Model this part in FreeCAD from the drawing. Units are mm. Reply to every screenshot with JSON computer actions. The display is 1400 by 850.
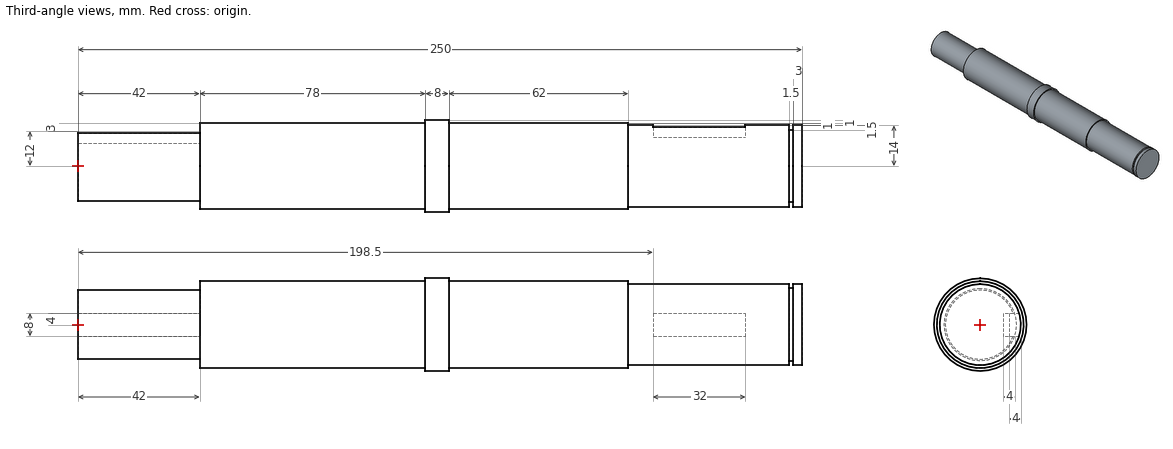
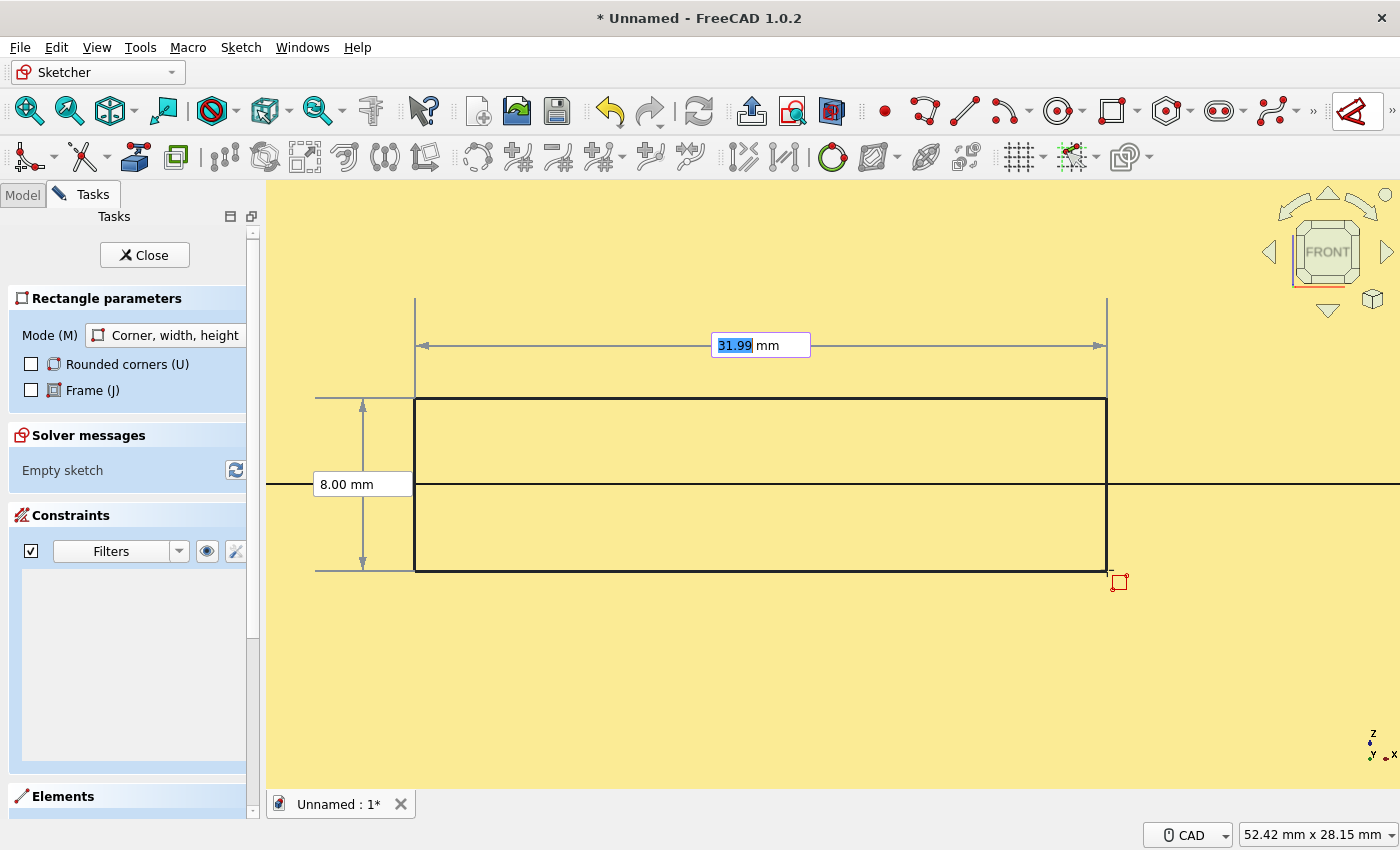
{"action": "type", "text": "32"}
{"action": "key", "text": "Tab"}
{"action": "type", "text": "8"}
{"action": "key", "text": "Return"}
{"action": "key", "text": "Escape"}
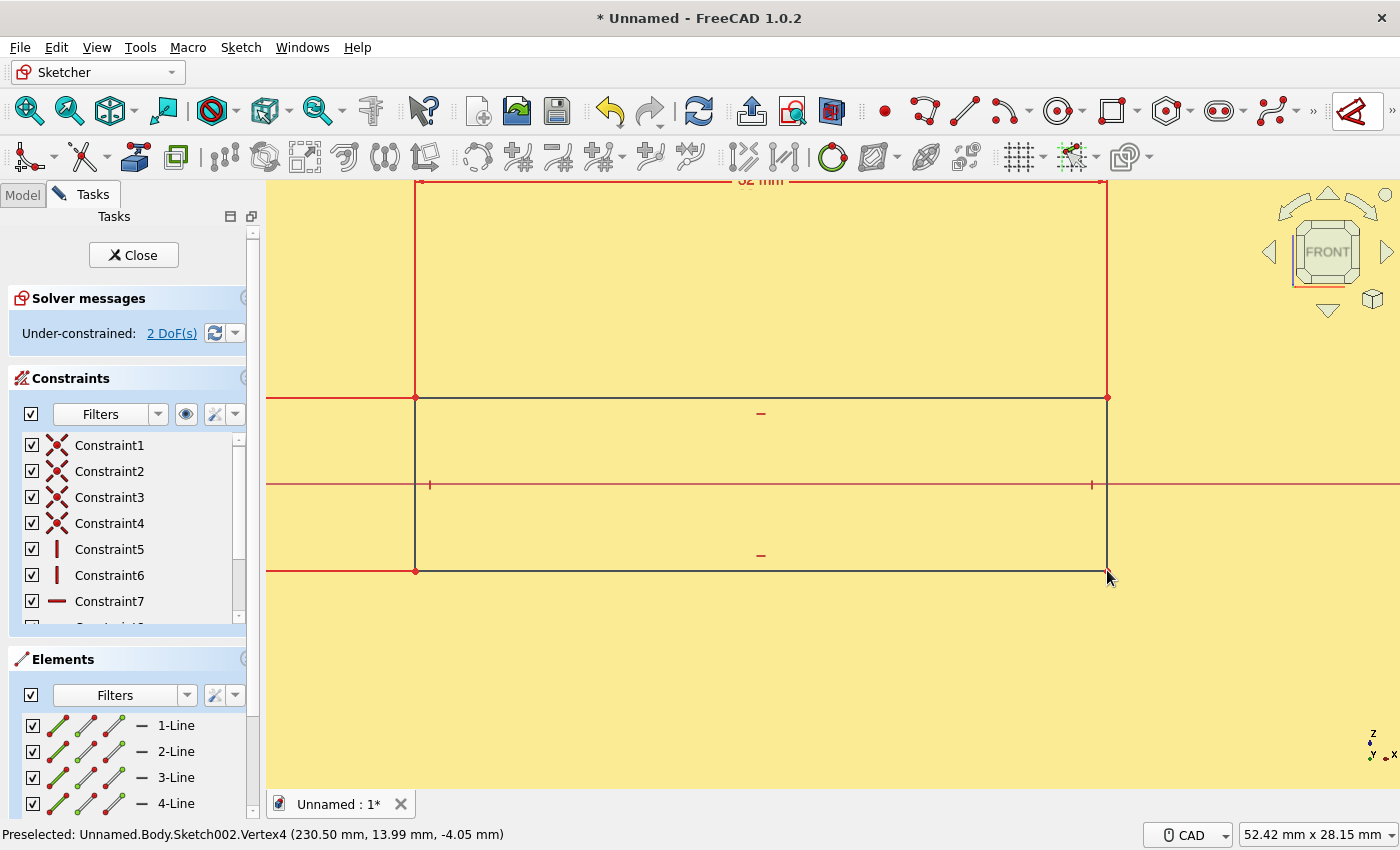
{"action": "left_click", "coordinate": [415, 398]}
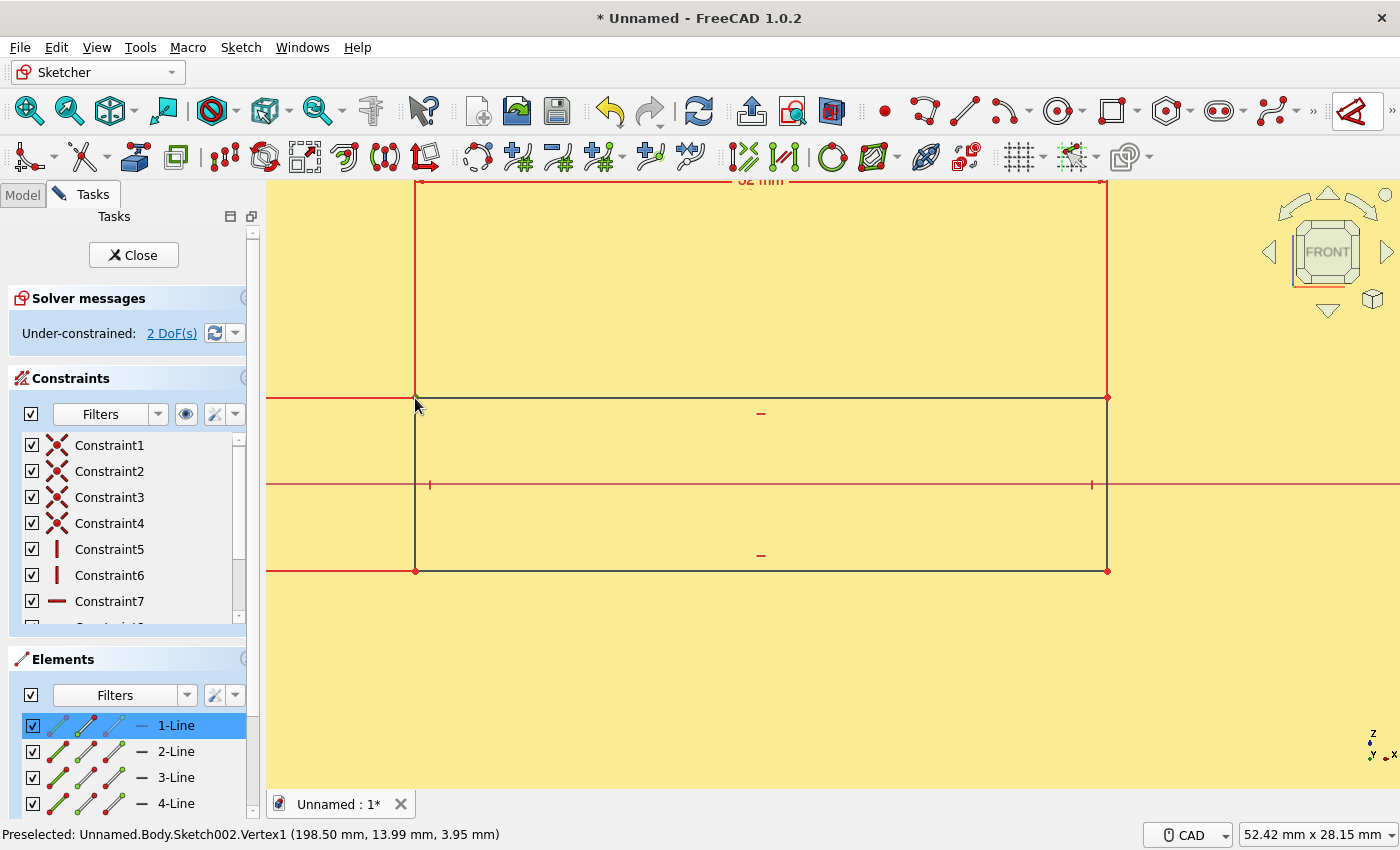
{"action": "left_click", "coordinate": [1378, 112]}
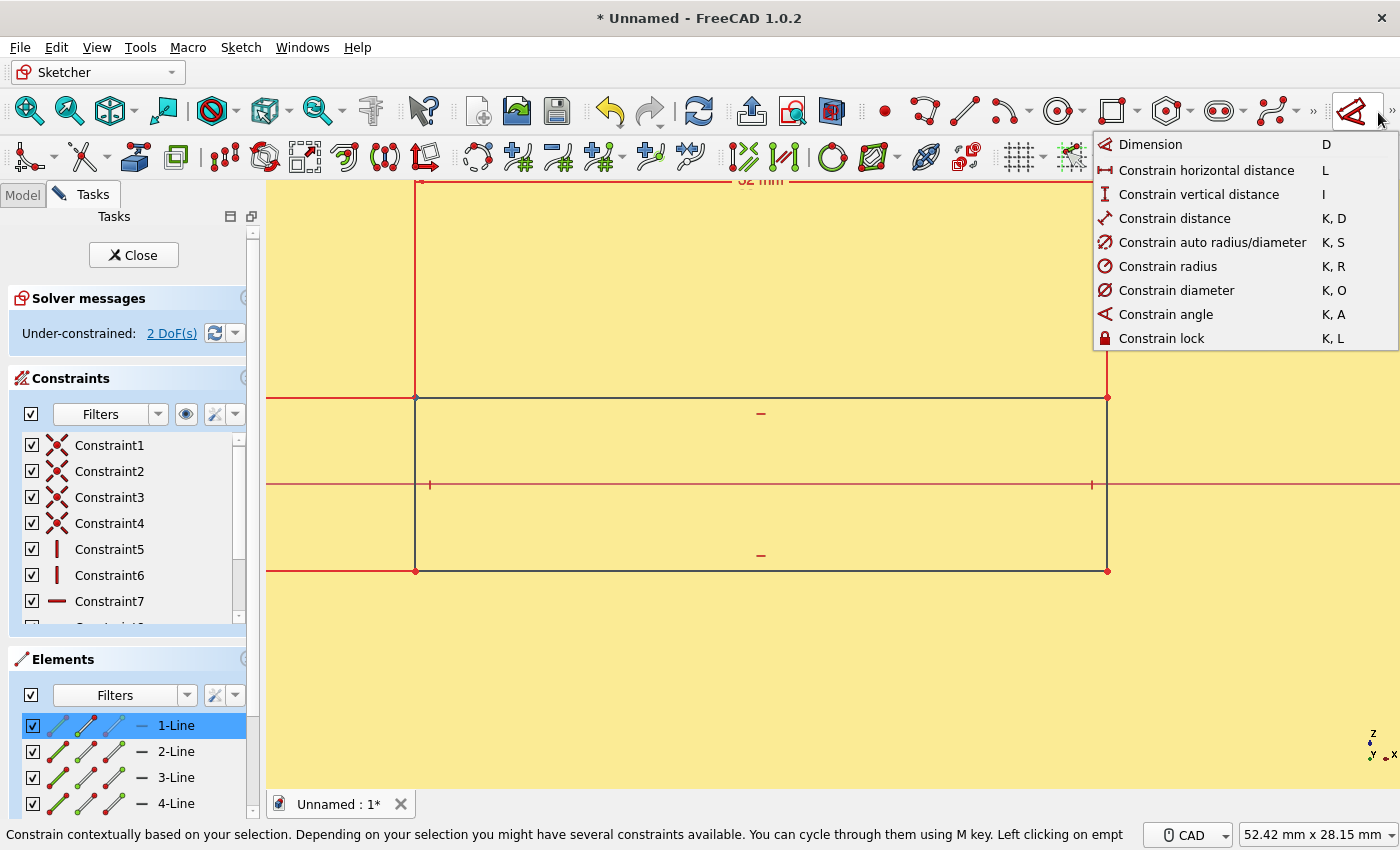
{"action": "left_click", "coordinate": [1246, 194]}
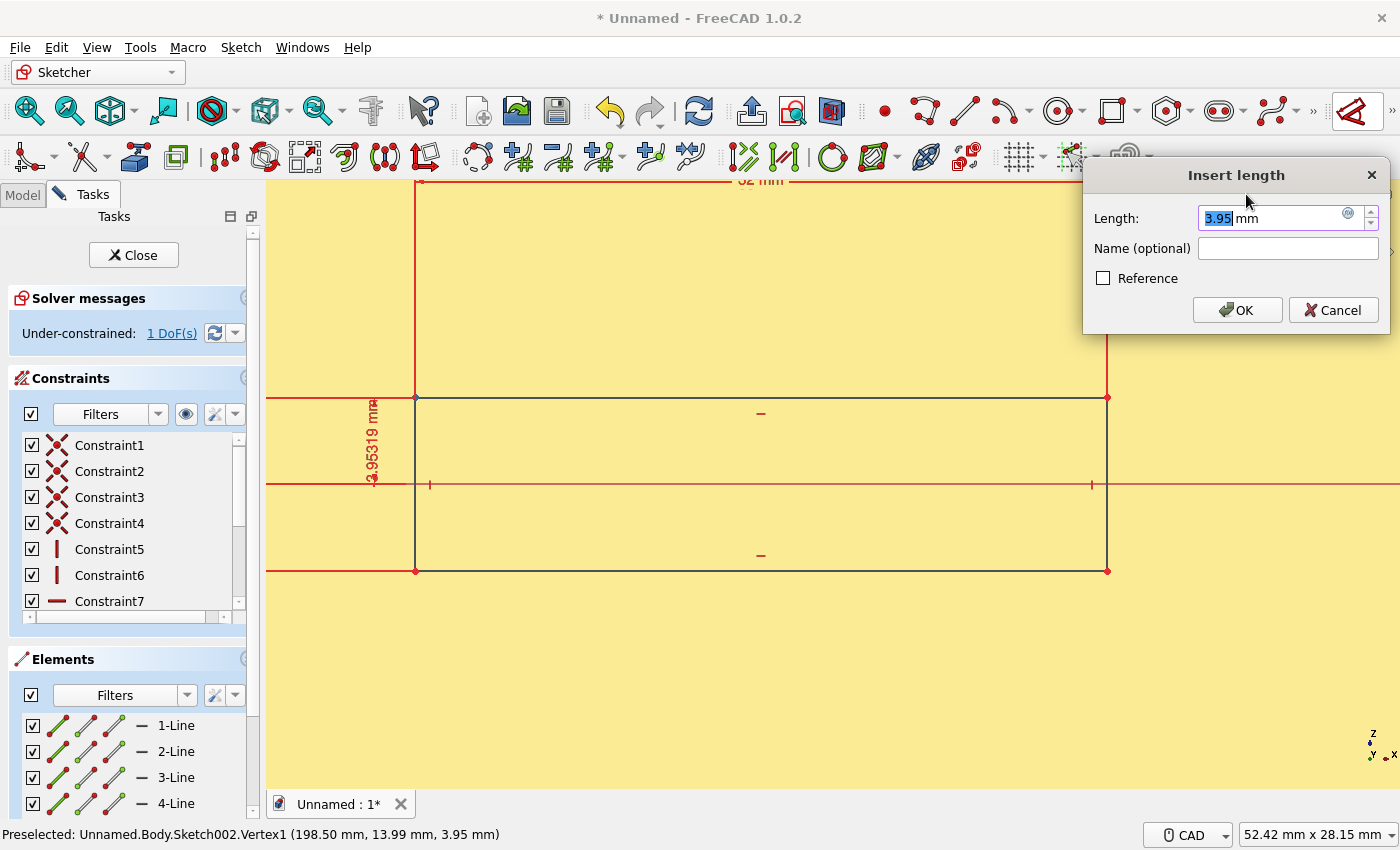
{"action": "type", "text": "4"}
{"action": "key", "text": "Return"}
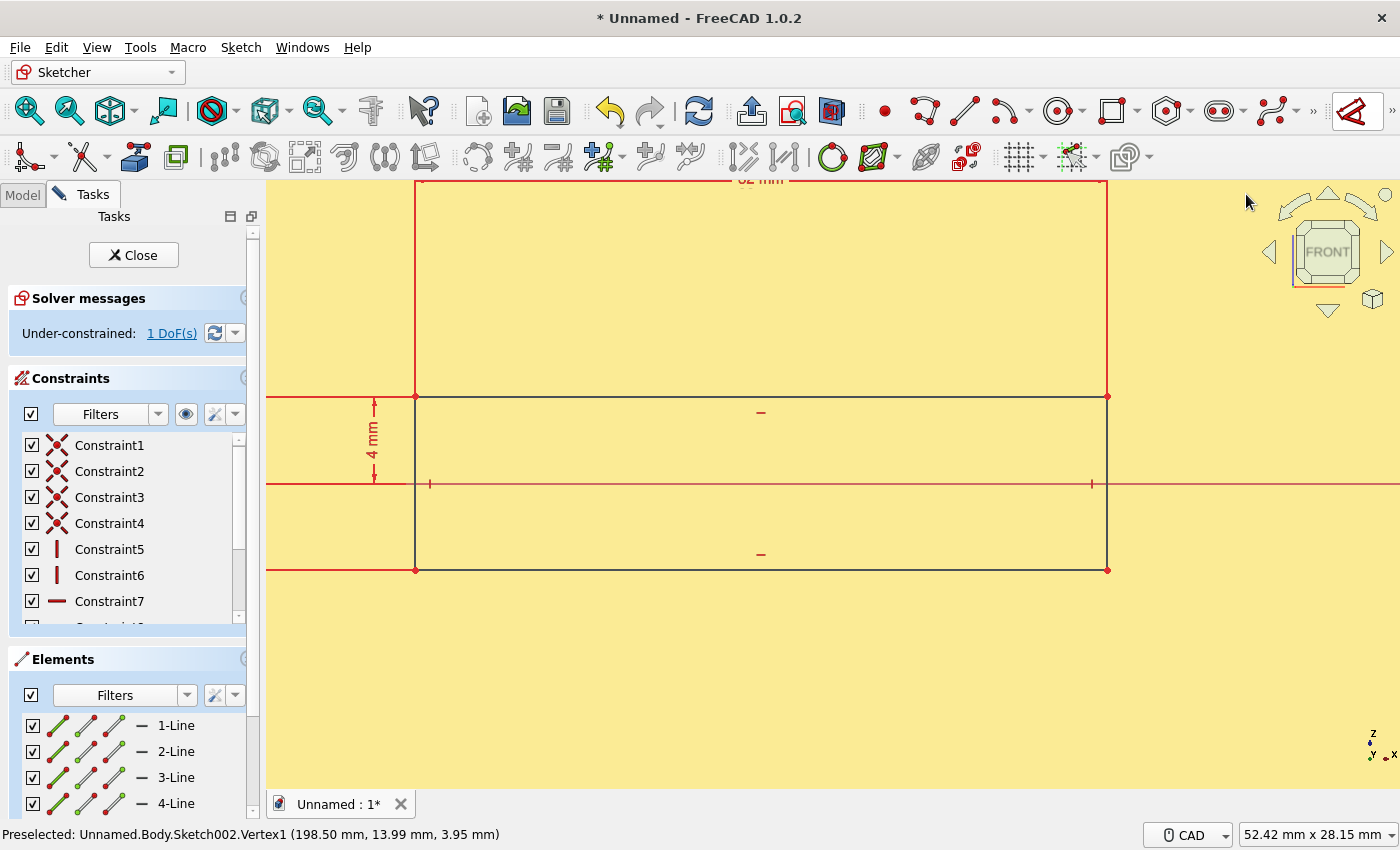
{"action": "left_click", "coordinate": [415, 397]}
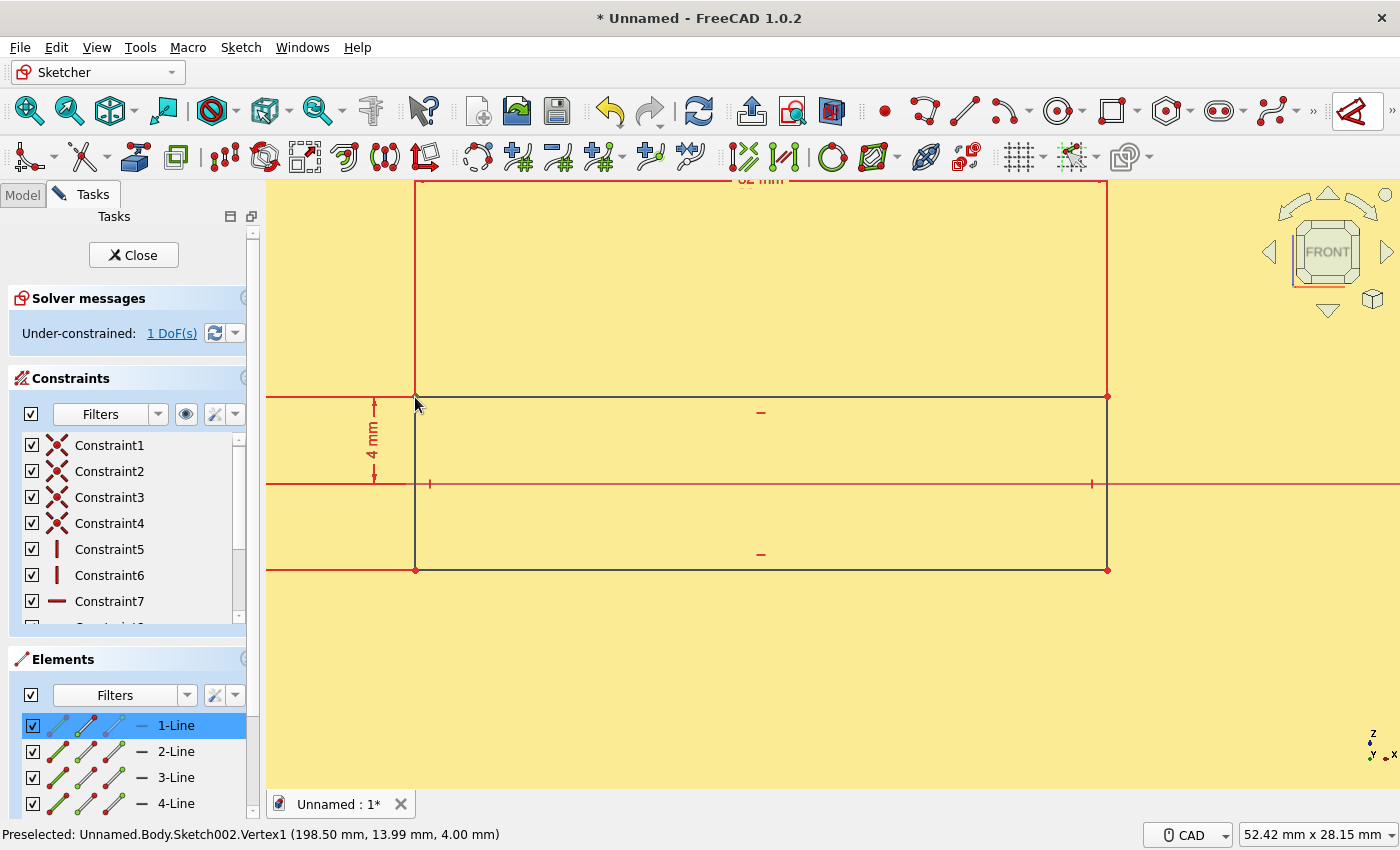
{"action": "left_click", "coordinate": [1378, 112]}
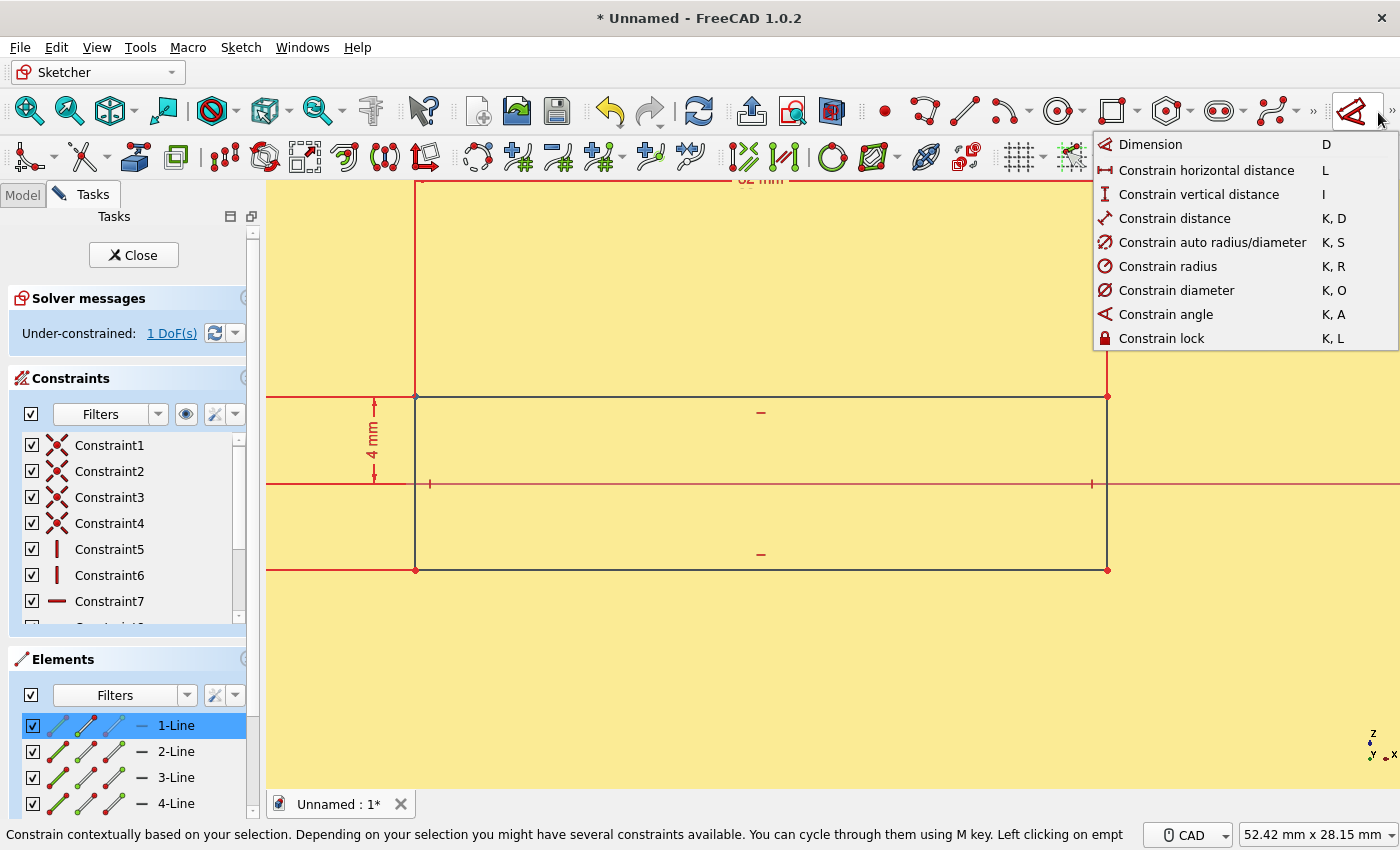
{"action": "left_click", "coordinate": [1246, 170]}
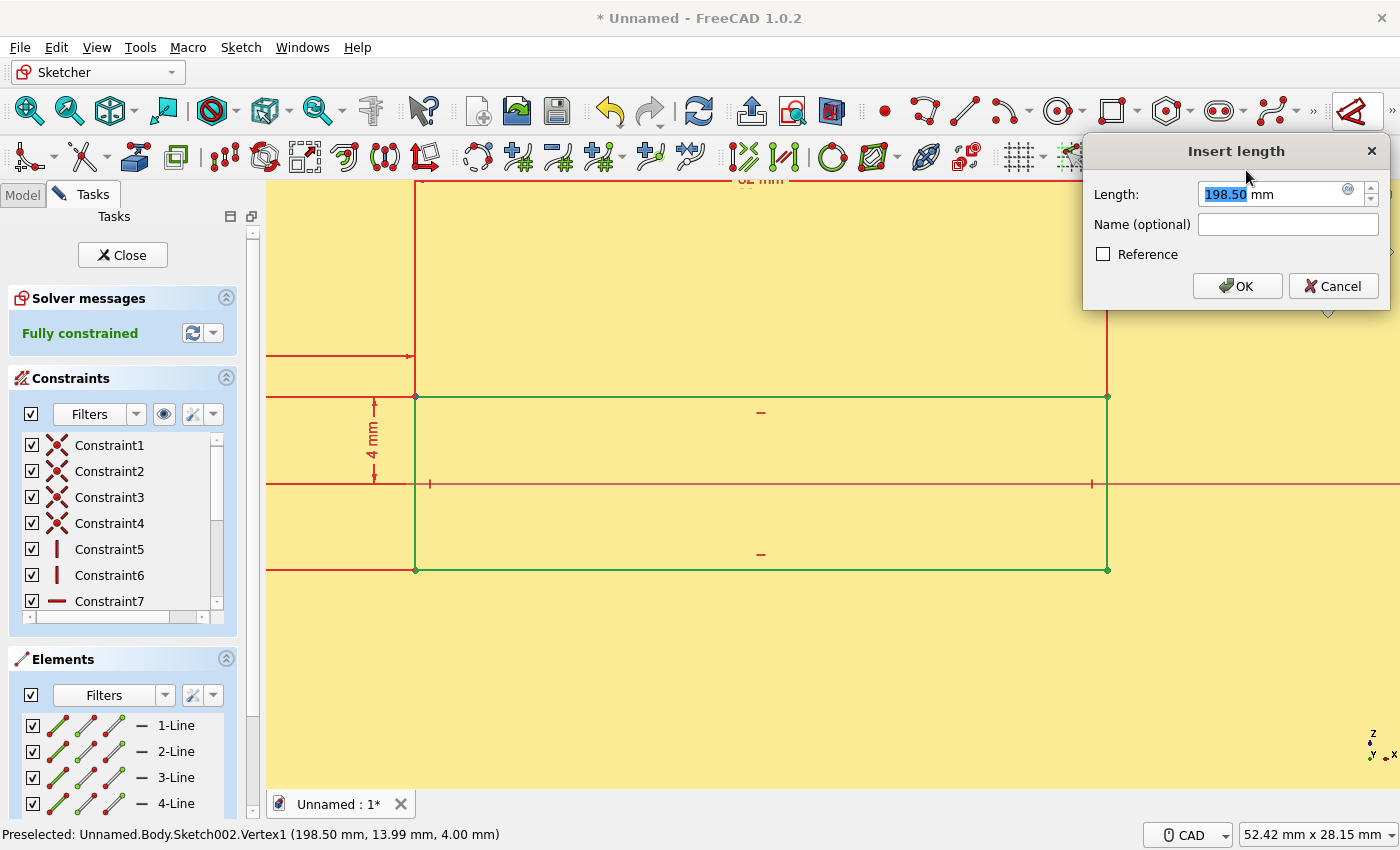
{"action": "type", "text": "198.5"}
{"action": "key", "text": "Return"}